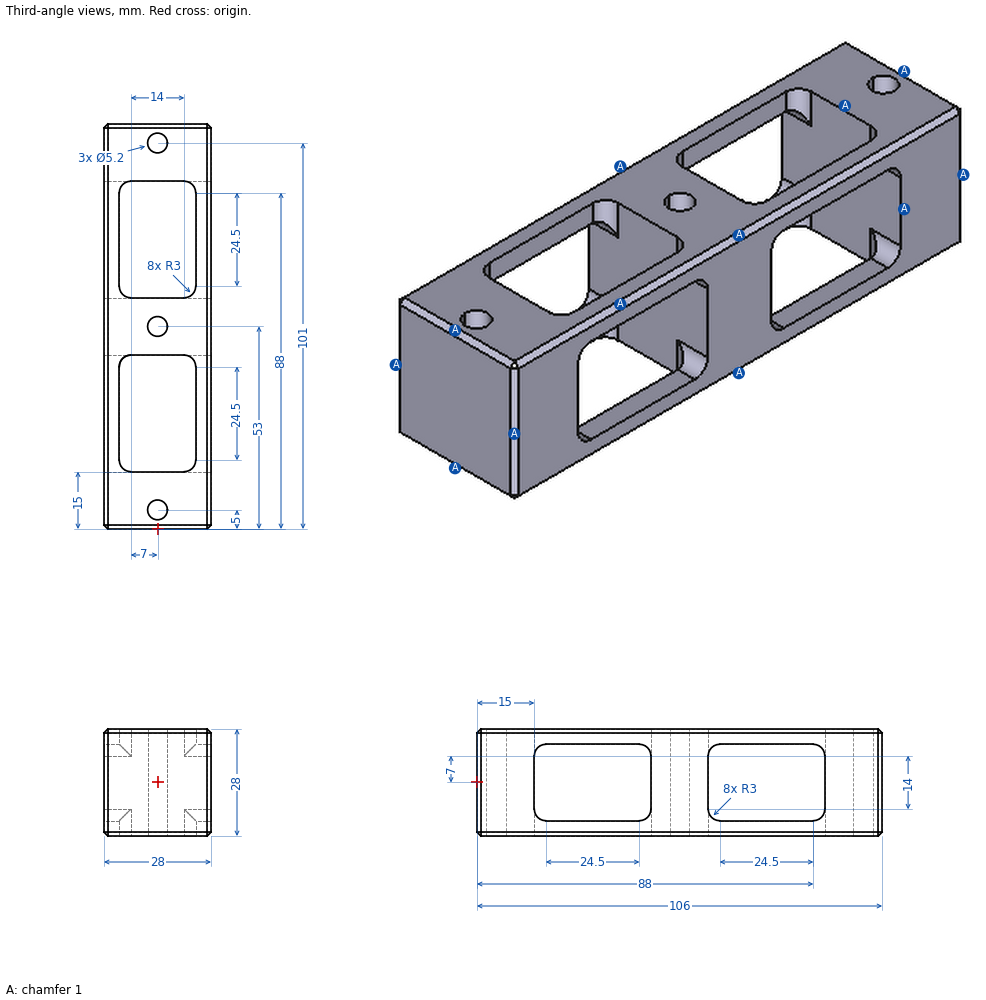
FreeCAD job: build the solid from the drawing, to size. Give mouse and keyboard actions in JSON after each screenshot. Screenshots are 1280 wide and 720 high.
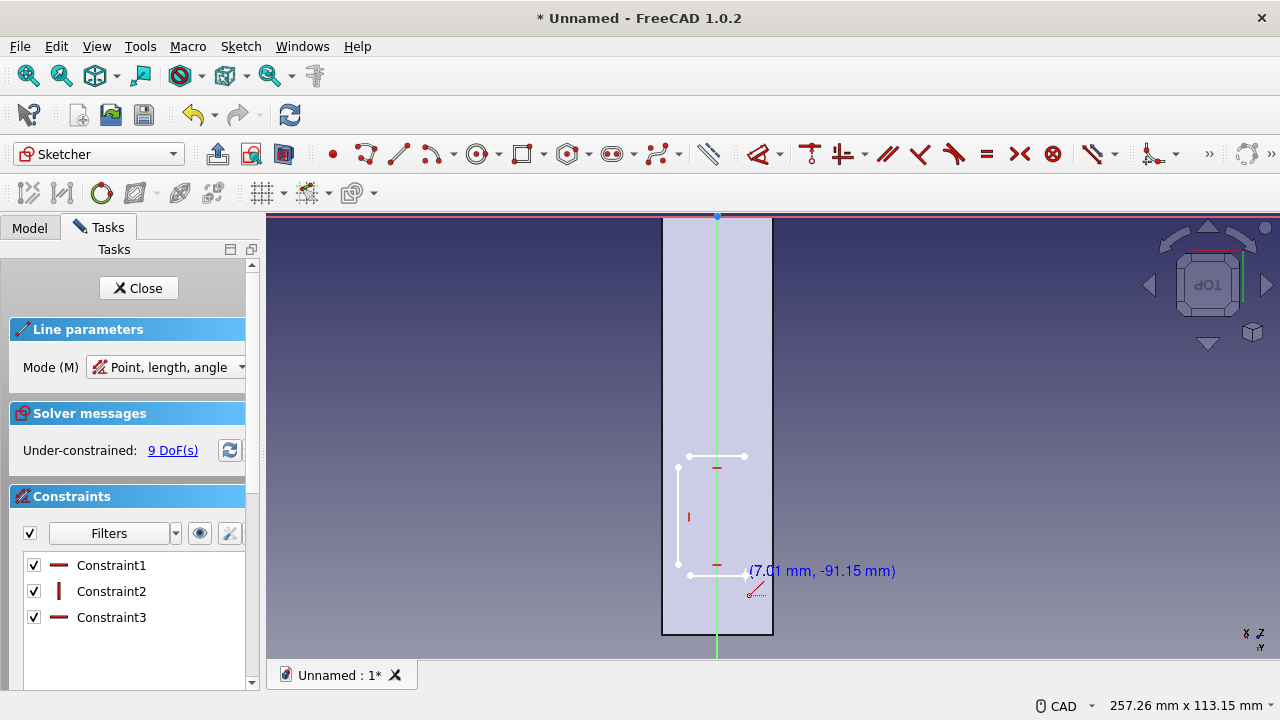
{"action": "left_click", "coordinate": [757, 564]}
{"action": "left_click", "coordinate": [757, 467]}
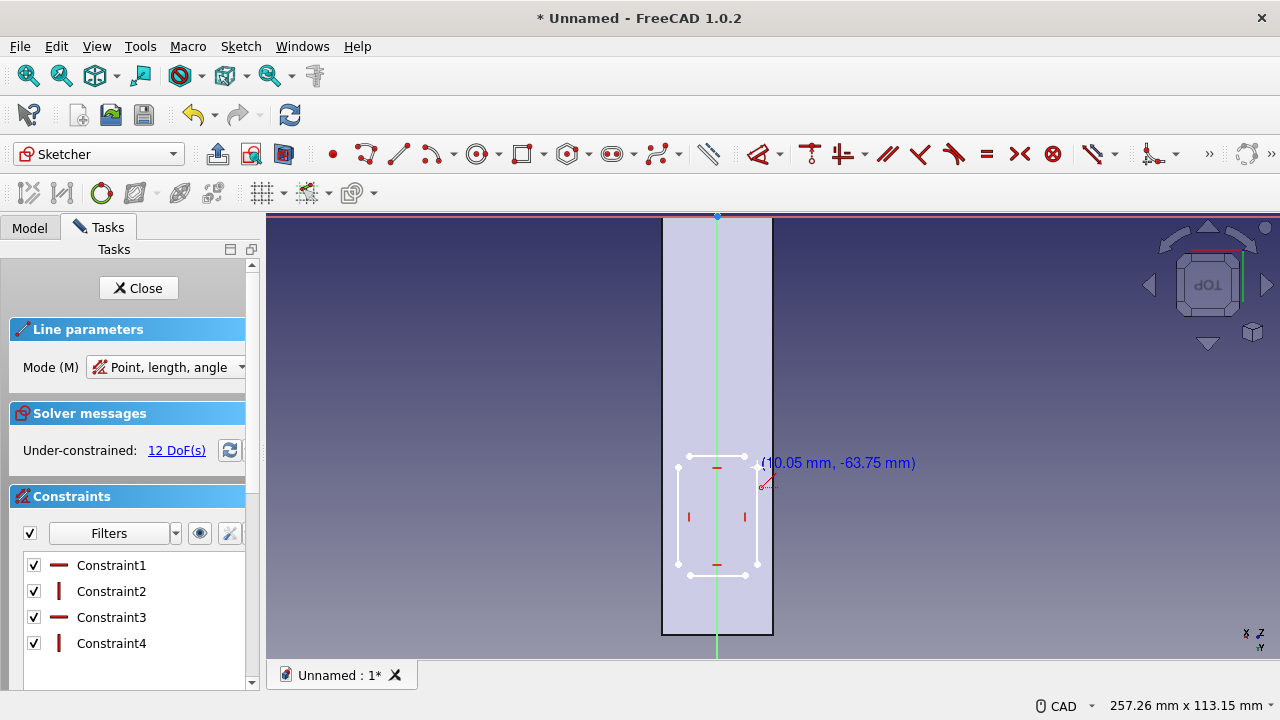
{"action": "left_click", "coordinate": [454, 154]}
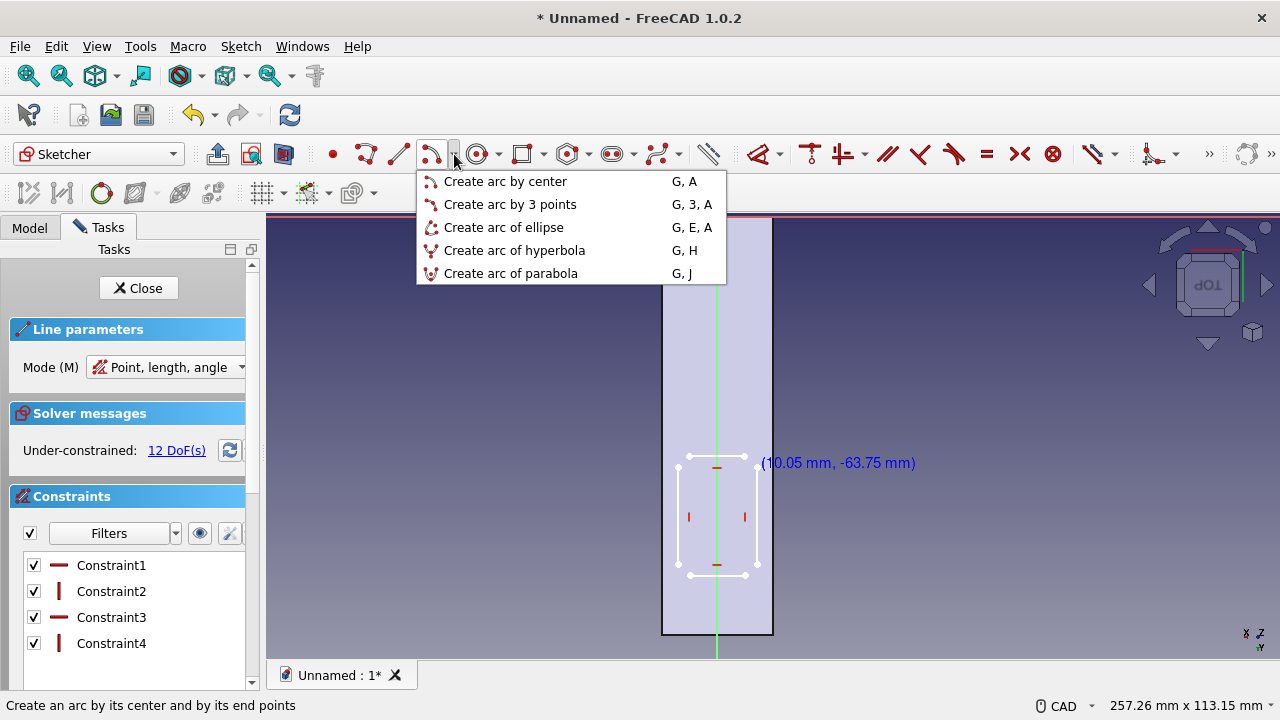
{"action": "left_click", "coordinate": [572, 204]}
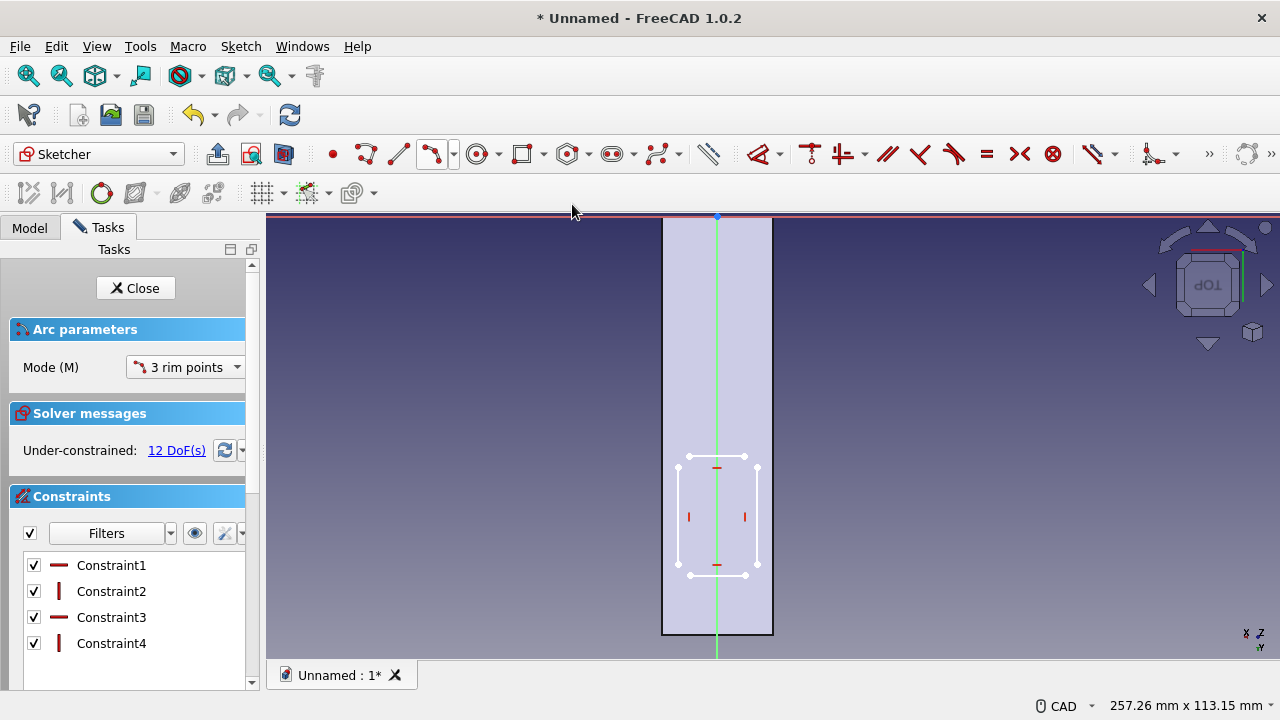
{"action": "left_click", "coordinate": [690, 456]}
{"action": "left_click", "coordinate": [678, 468]}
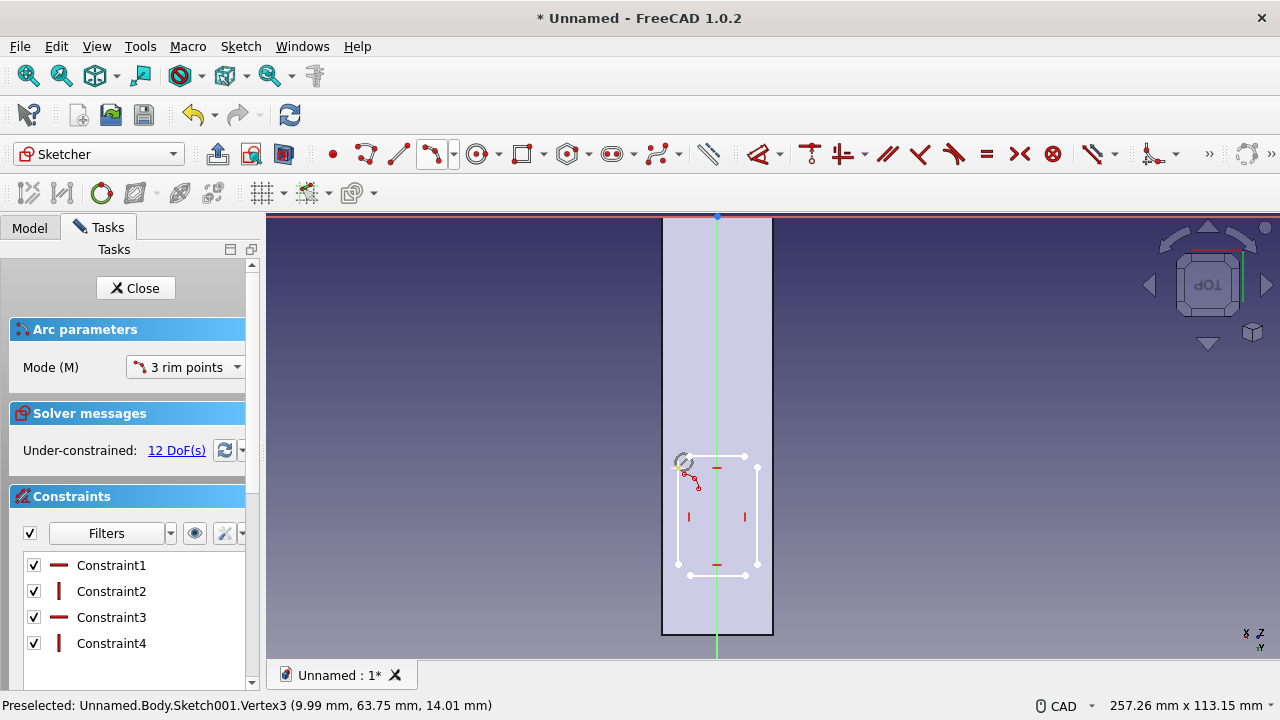
{"action": "scroll", "coordinate": [681, 459], "scroll_direction": "up", "scroll_amount": 8}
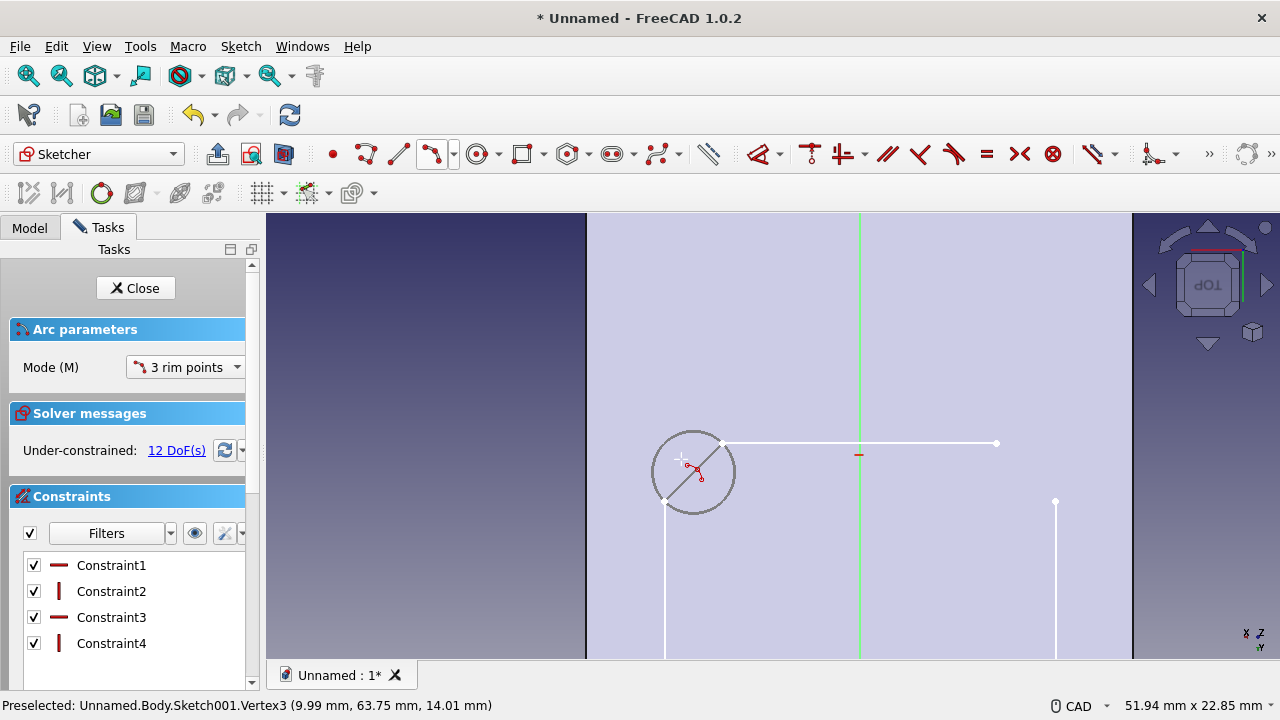
{"action": "left_click", "coordinate": [681, 455]}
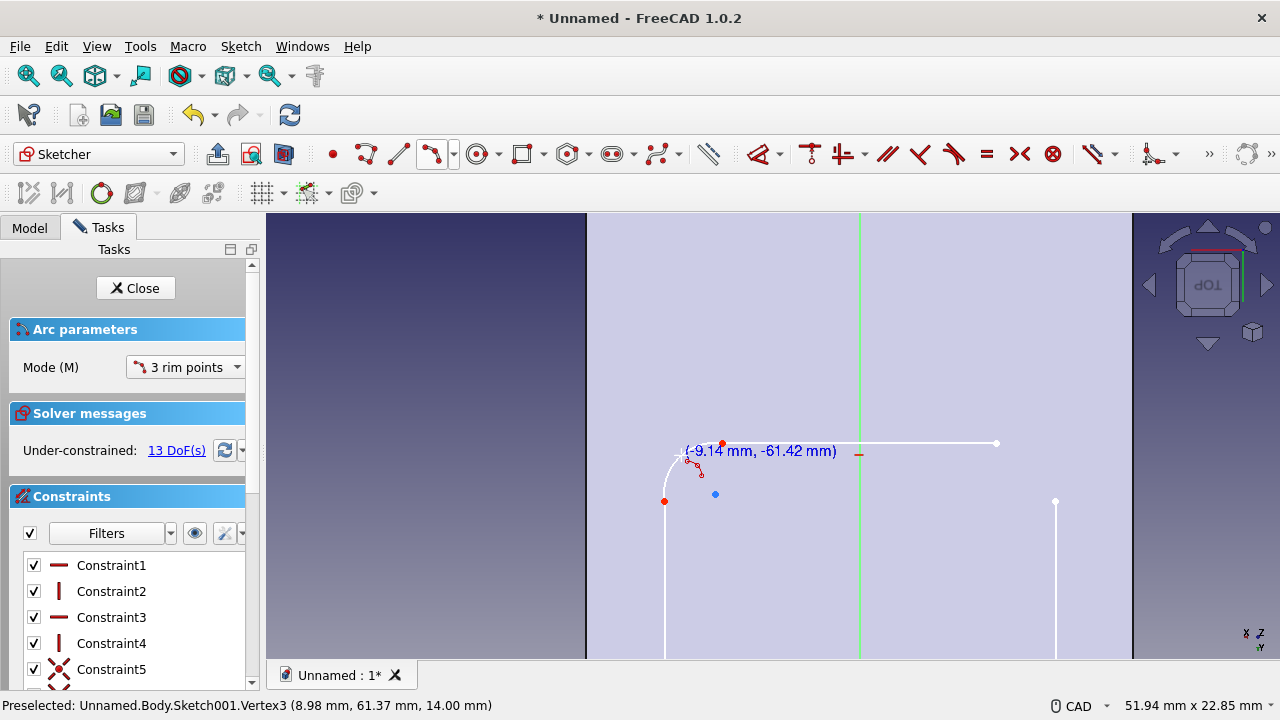
{"action": "scroll", "coordinate": [680, 462], "scroll_direction": "down", "scroll_amount": 10}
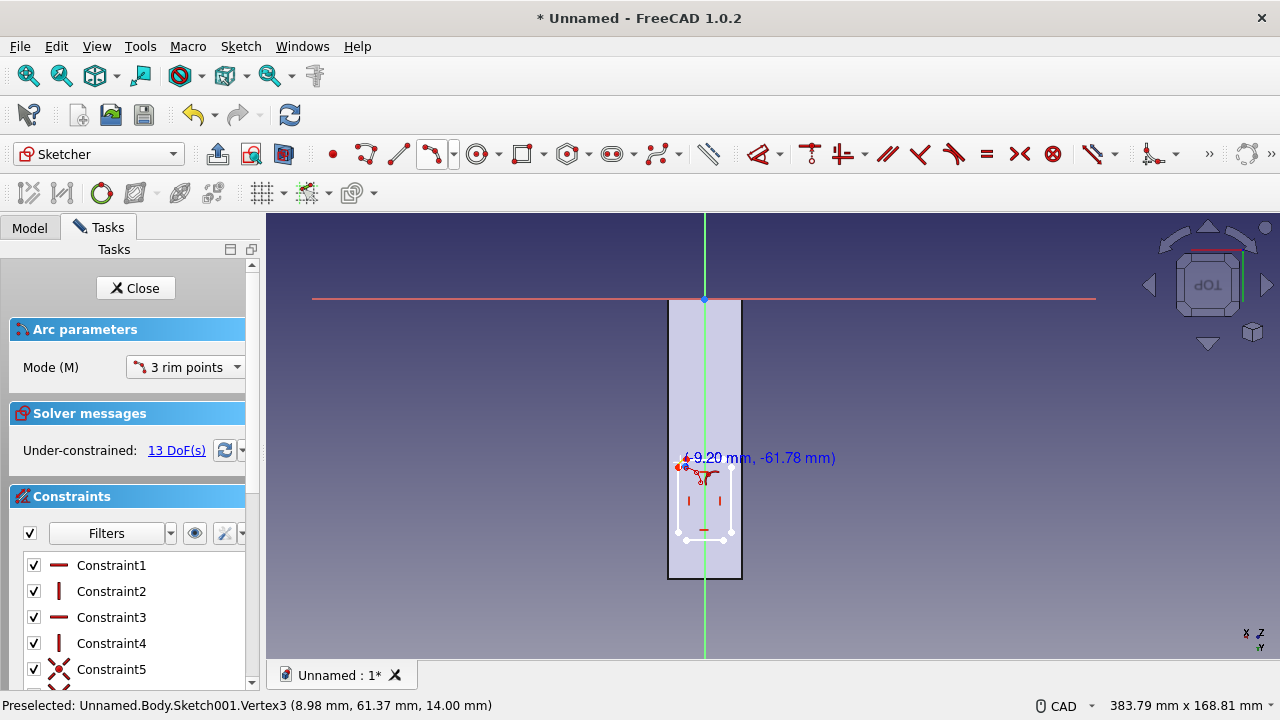
{"action": "scroll", "coordinate": [678, 532], "scroll_direction": "up", "scroll_amount": 2}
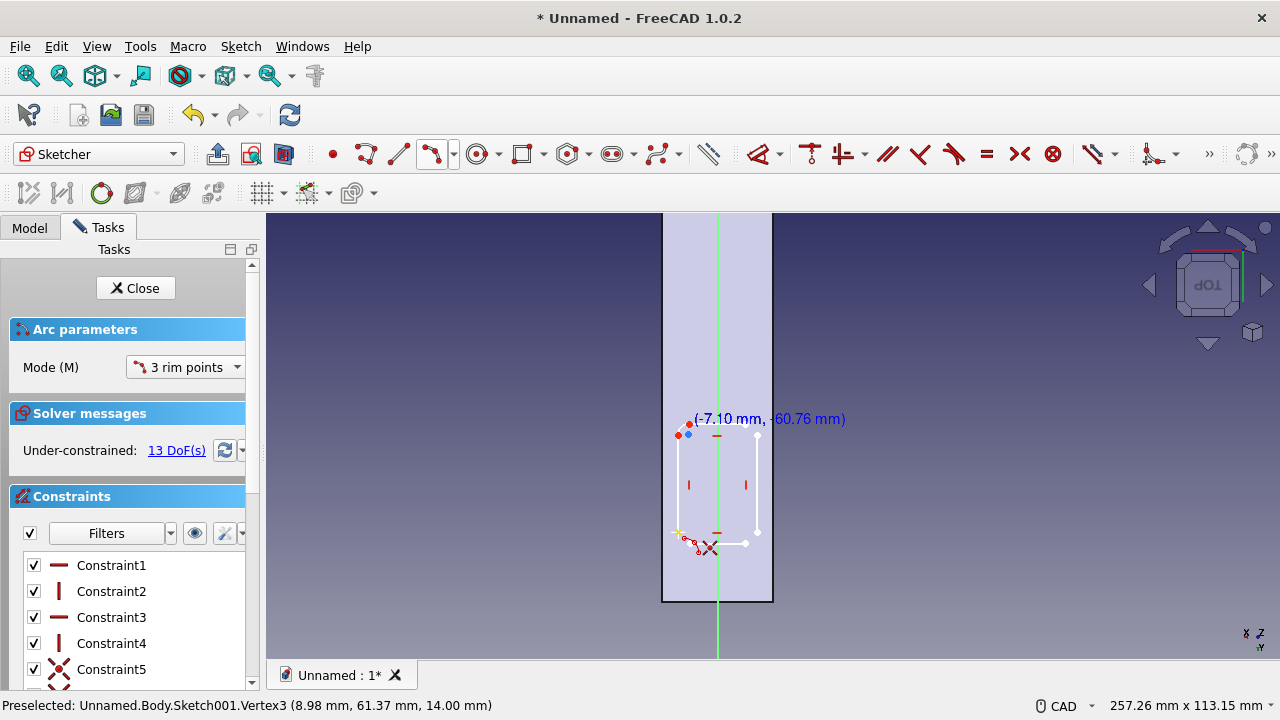
{"action": "left_click", "coordinate": [678, 533]}
{"action": "left_click", "coordinate": [690, 544]}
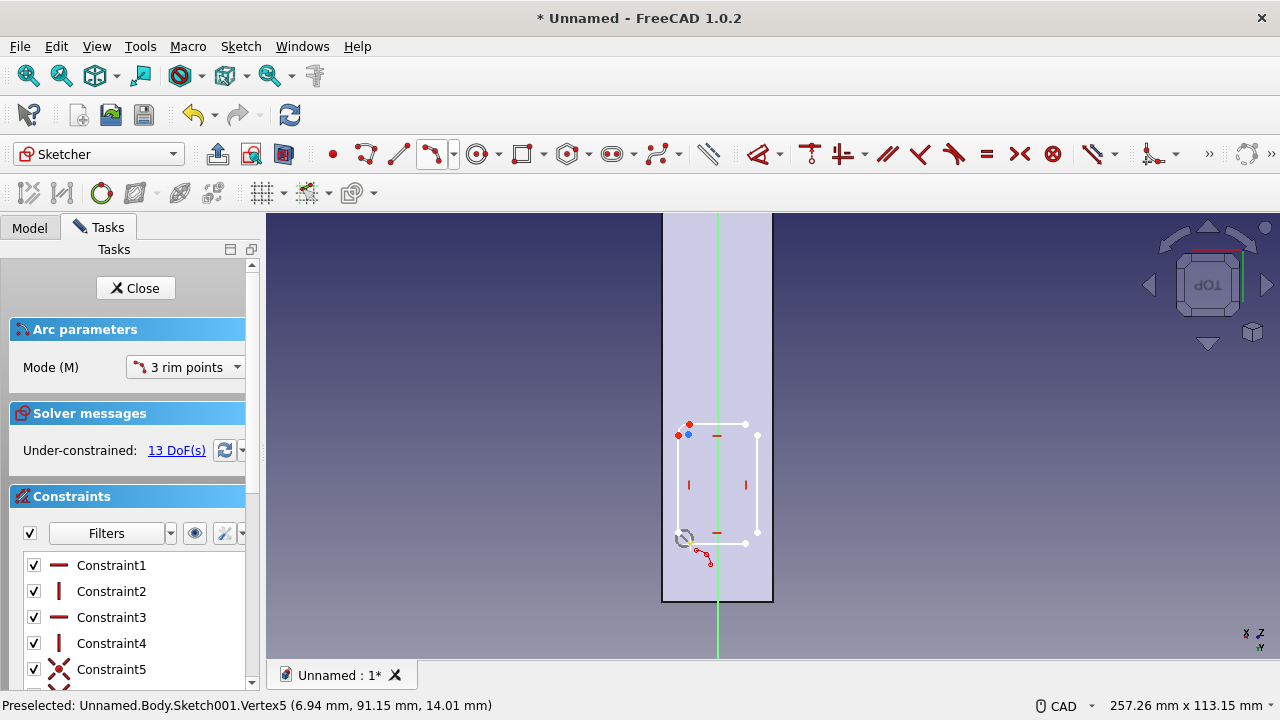
{"action": "scroll", "coordinate": [682, 540], "scroll_direction": "up", "scroll_amount": 8}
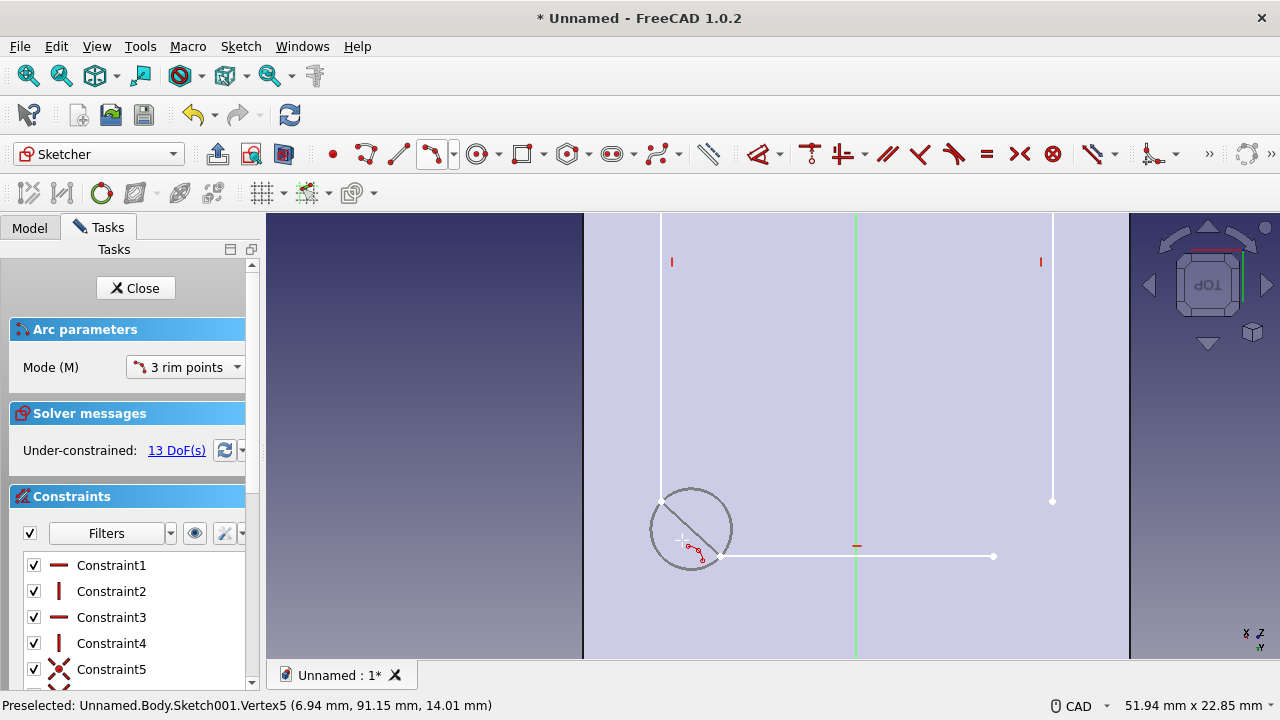
{"action": "left_click", "coordinate": [678, 536]}